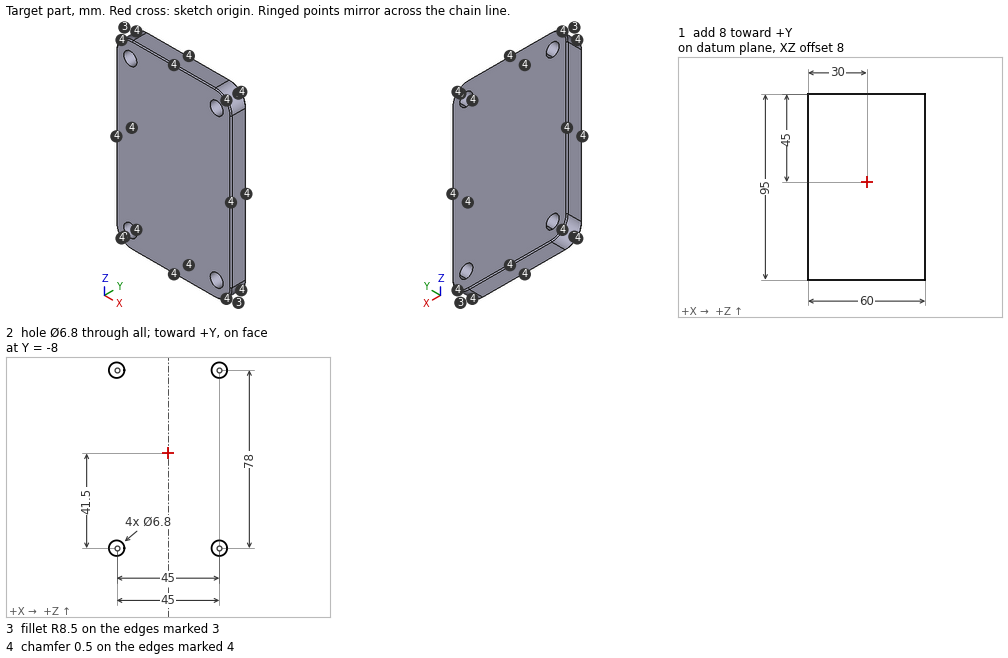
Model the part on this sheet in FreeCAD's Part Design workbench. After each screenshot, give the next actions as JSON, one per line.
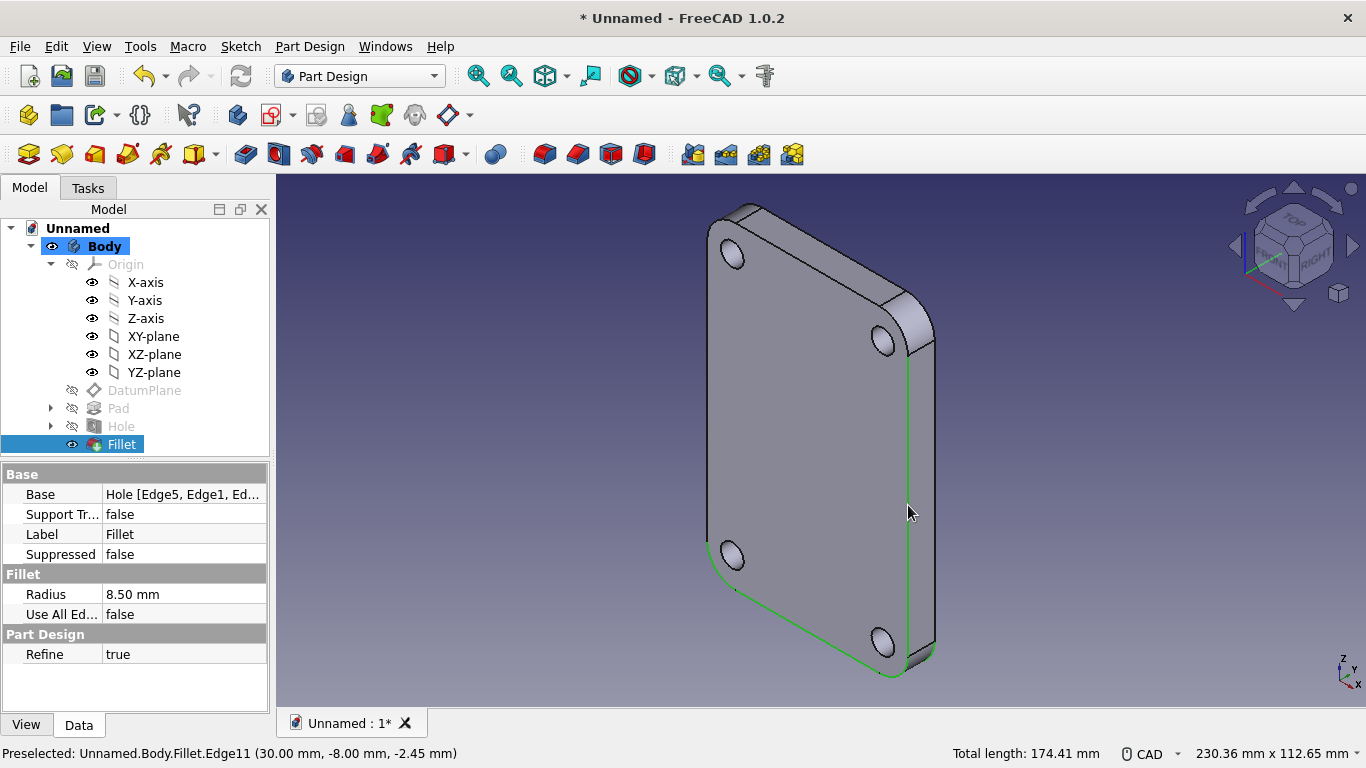
{"action": "left_click", "coordinate": [808, 264], "text": "ctrl"}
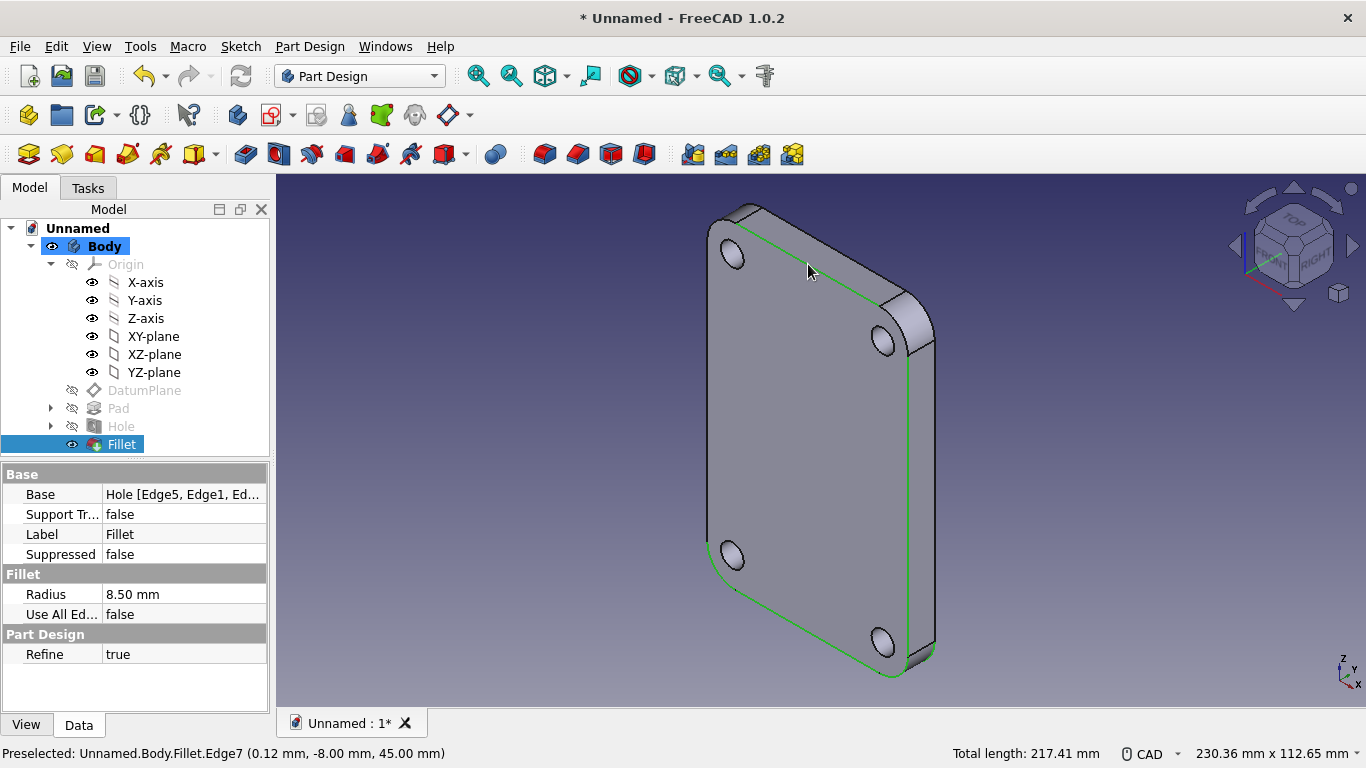
{"action": "left_click", "coordinate": [713, 222], "text": "ctrl"}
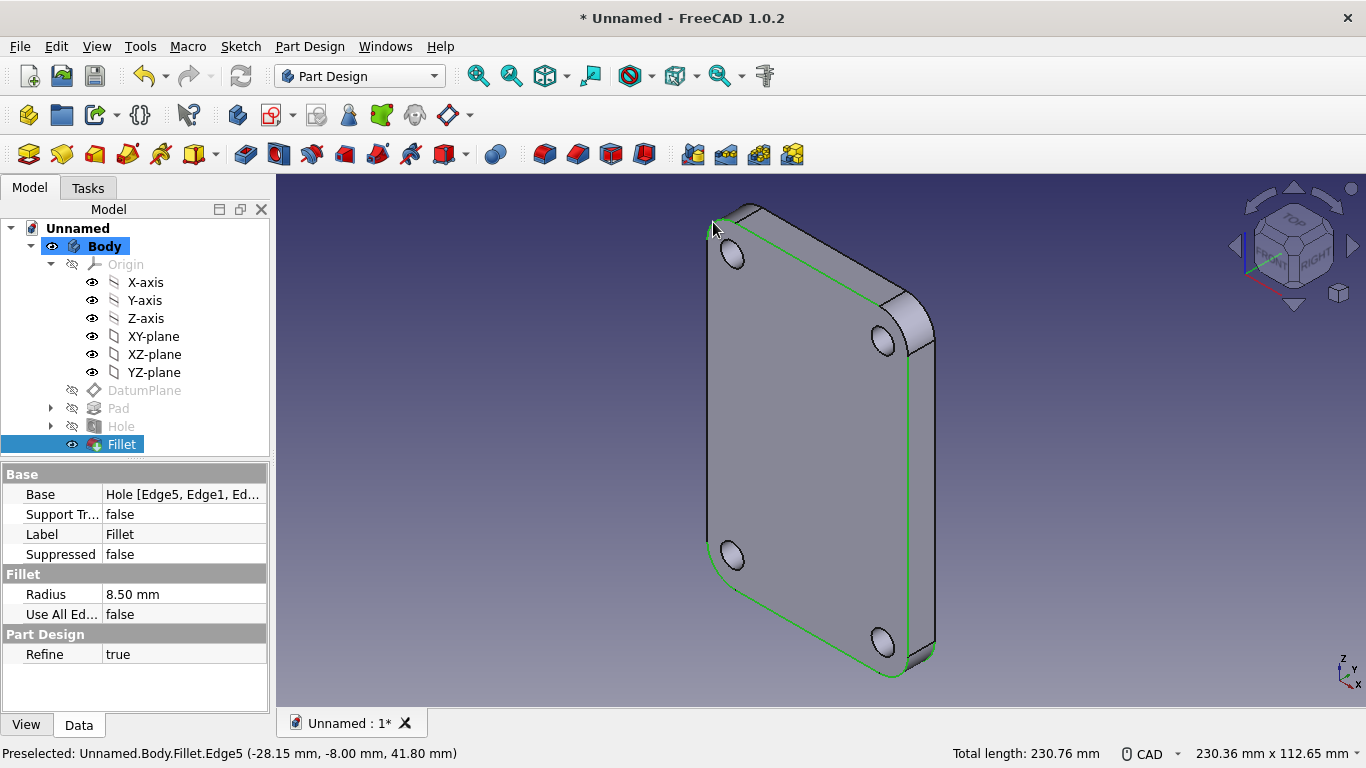
{"action": "left_click", "coordinate": [900, 326], "text": "ctrl"}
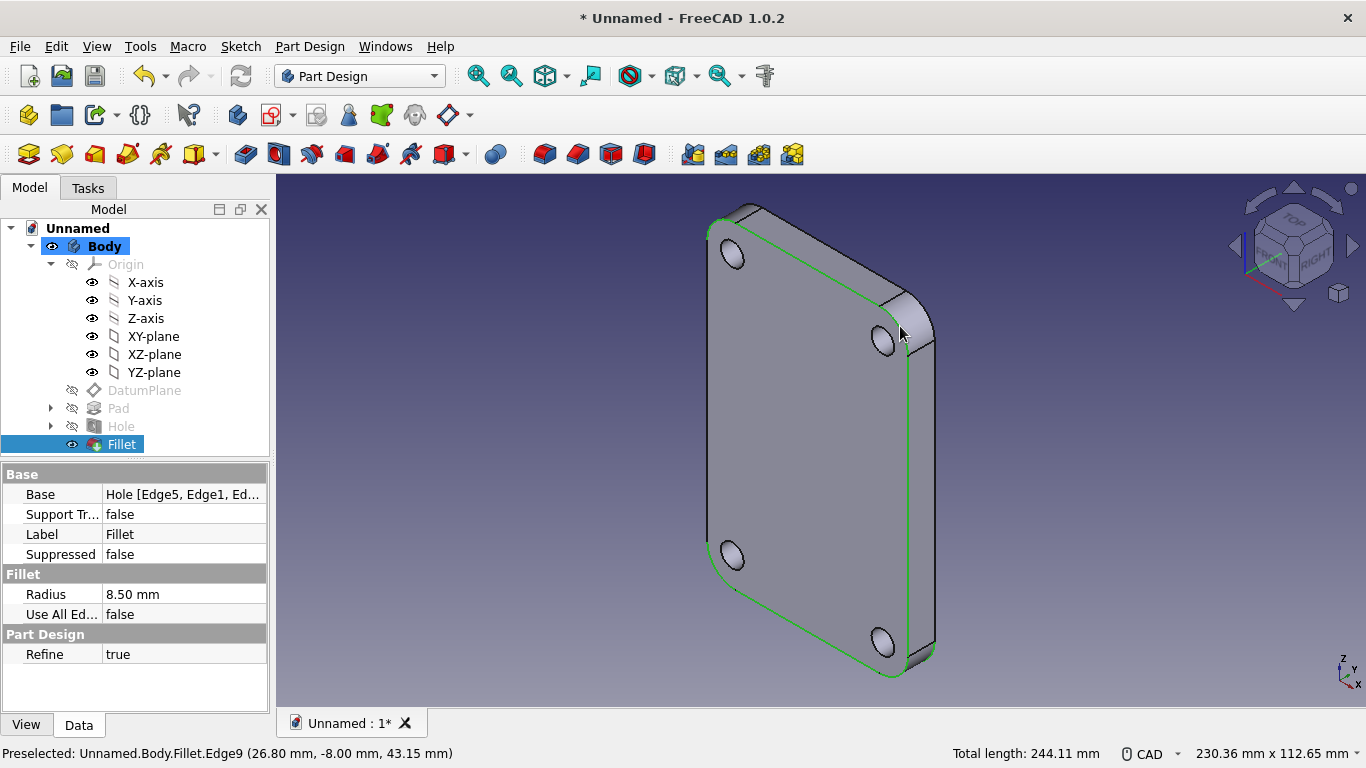
{"action": "left_click", "coordinate": [754, 203], "text": "ctrl"}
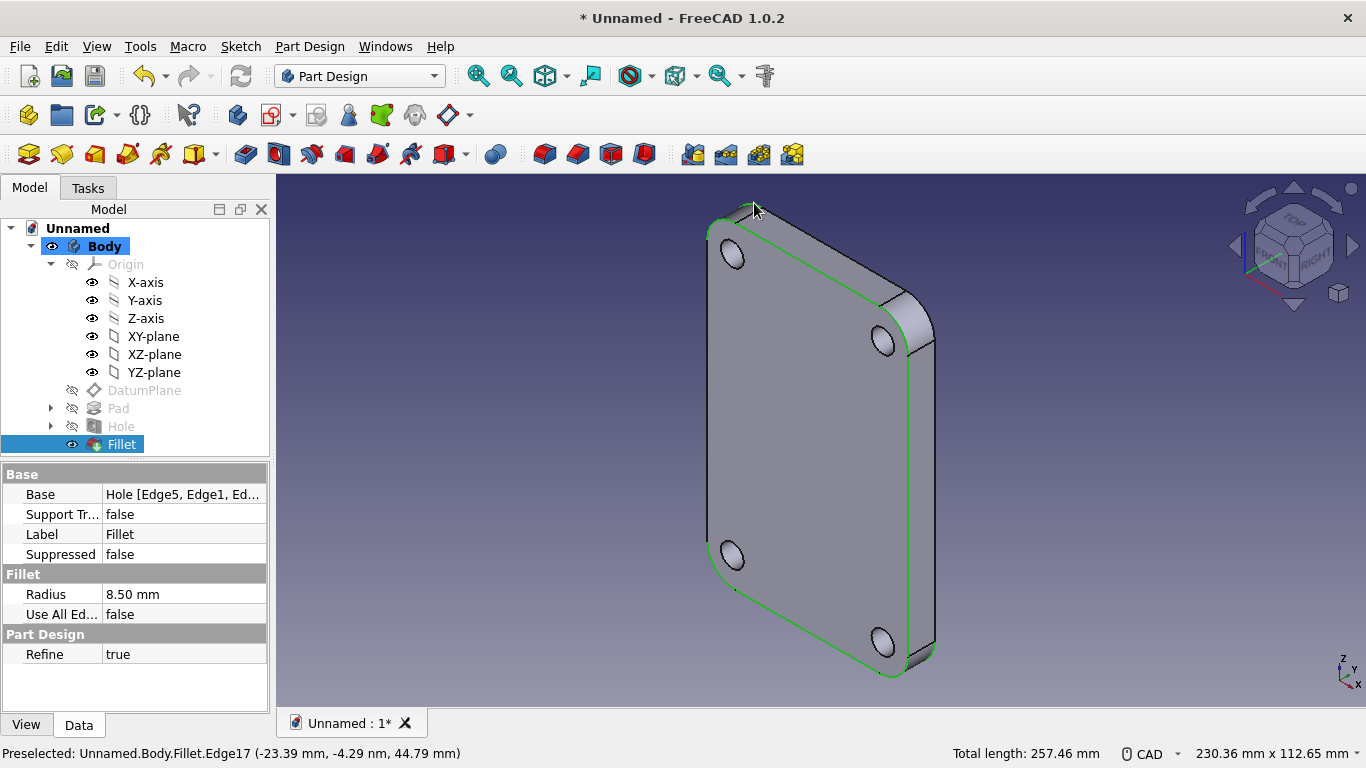
{"action": "left_click", "coordinate": [912, 293], "text": "ctrl"}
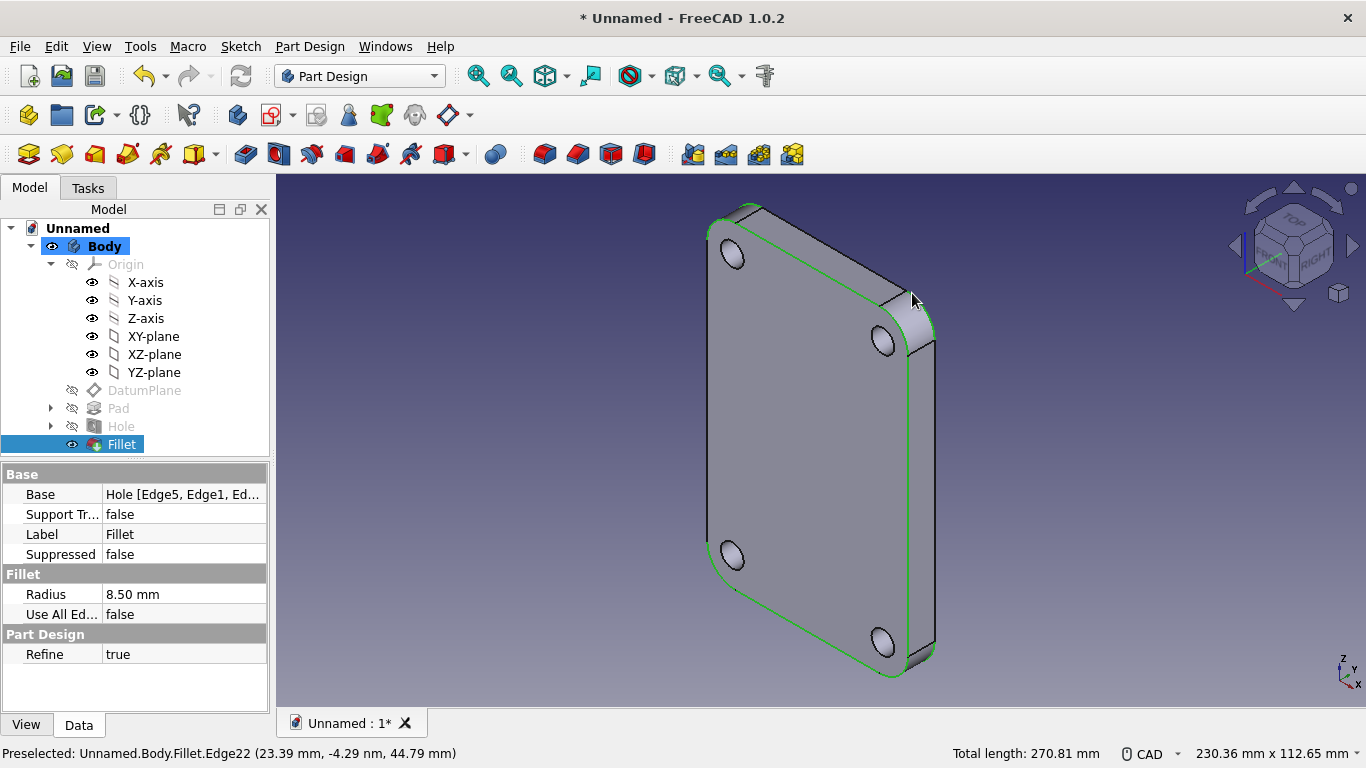
{"action": "key", "text": "2"}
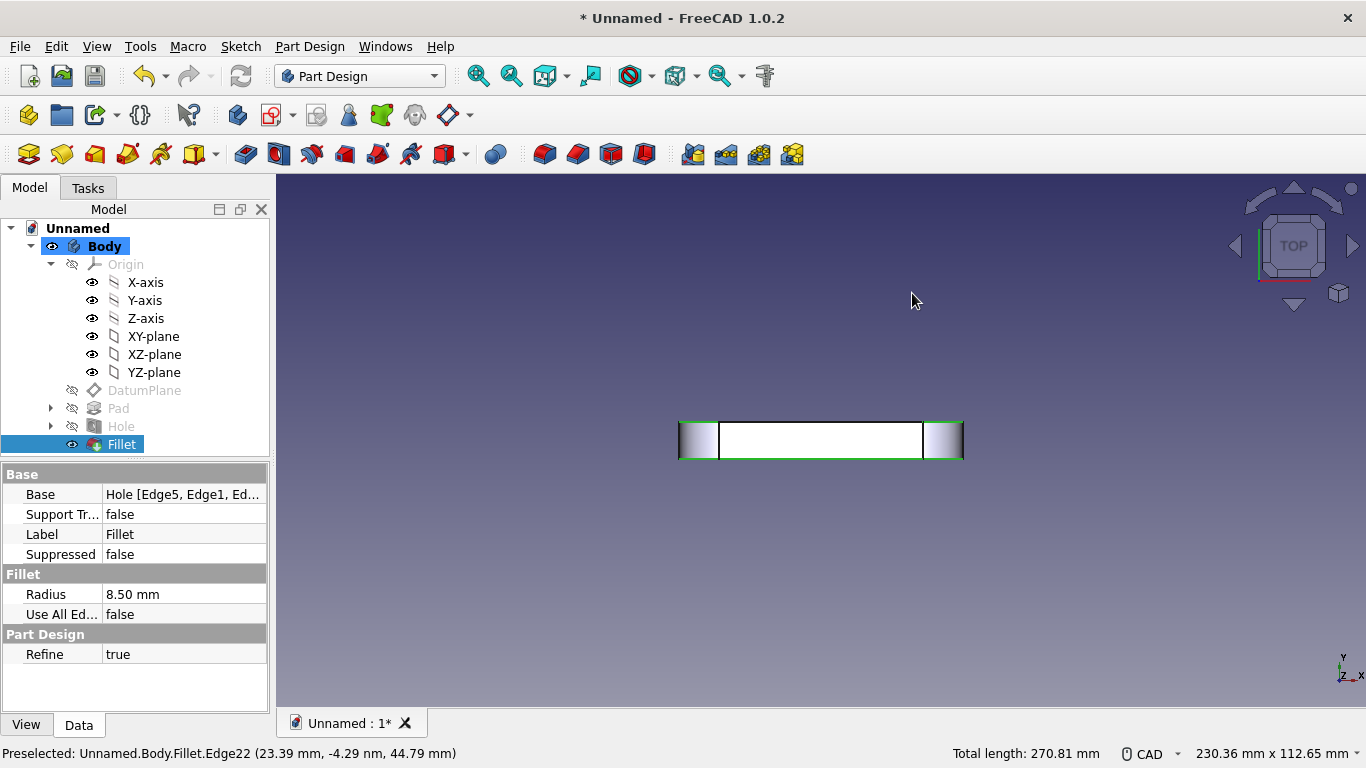
{"action": "left_click", "coordinate": [479, 76]}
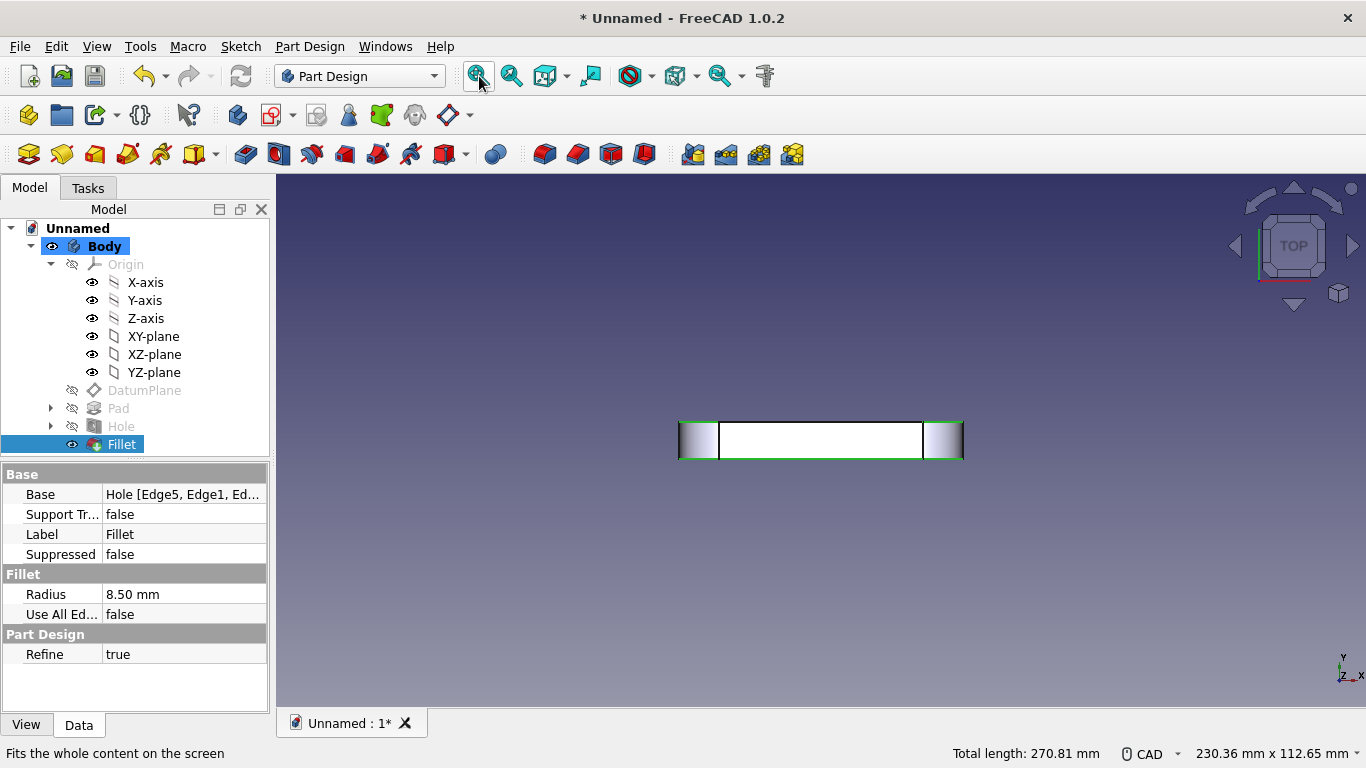
{"action": "left_click", "coordinate": [821, 421], "text": "ctrl"}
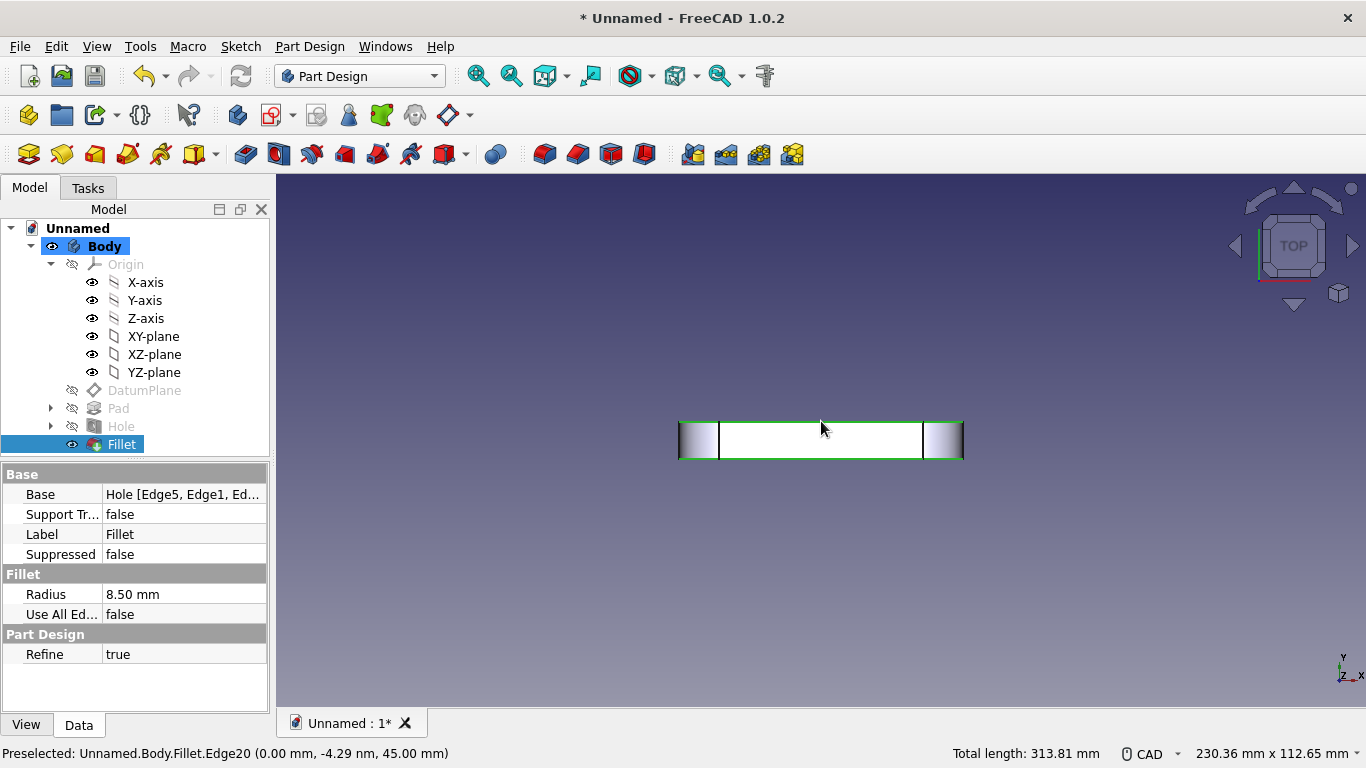
{"action": "key", "text": "1"}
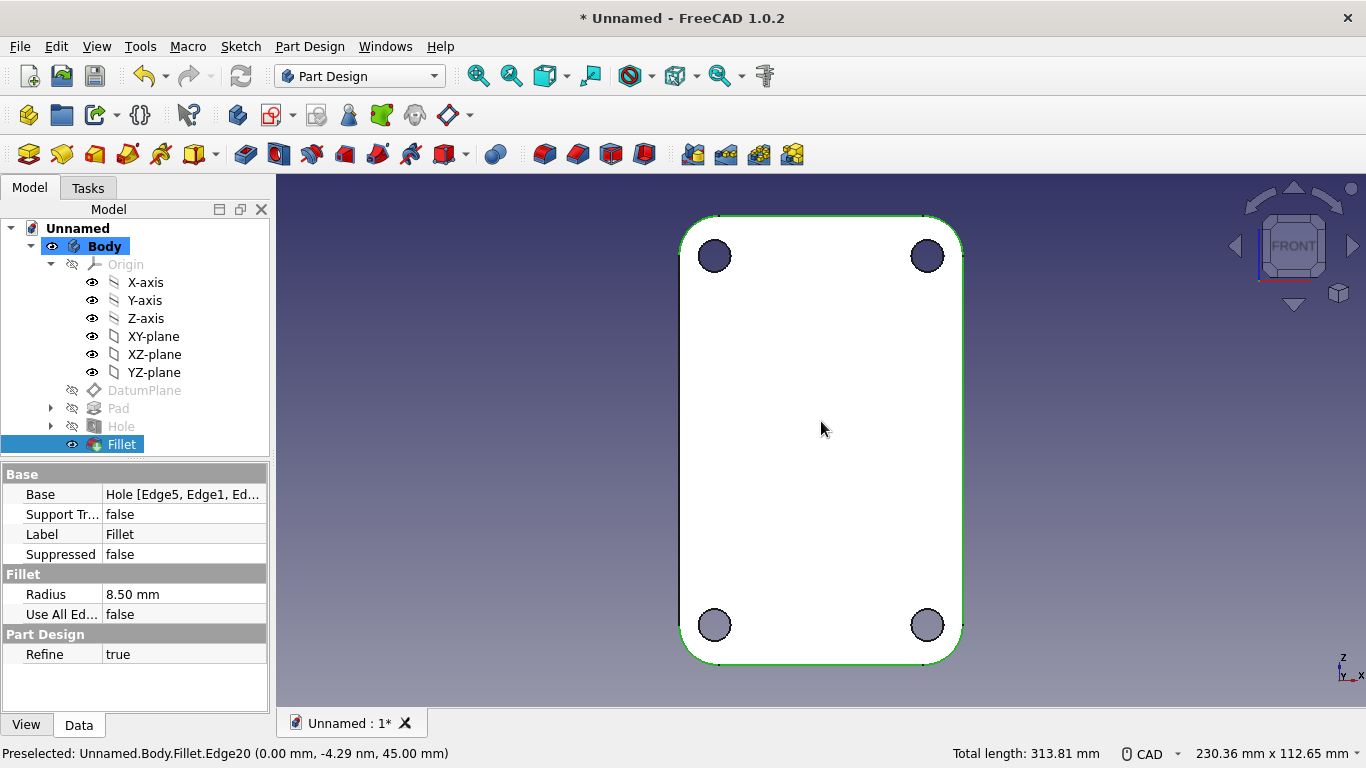
{"action": "left_click", "coordinate": [679, 439], "text": "ctrl"}